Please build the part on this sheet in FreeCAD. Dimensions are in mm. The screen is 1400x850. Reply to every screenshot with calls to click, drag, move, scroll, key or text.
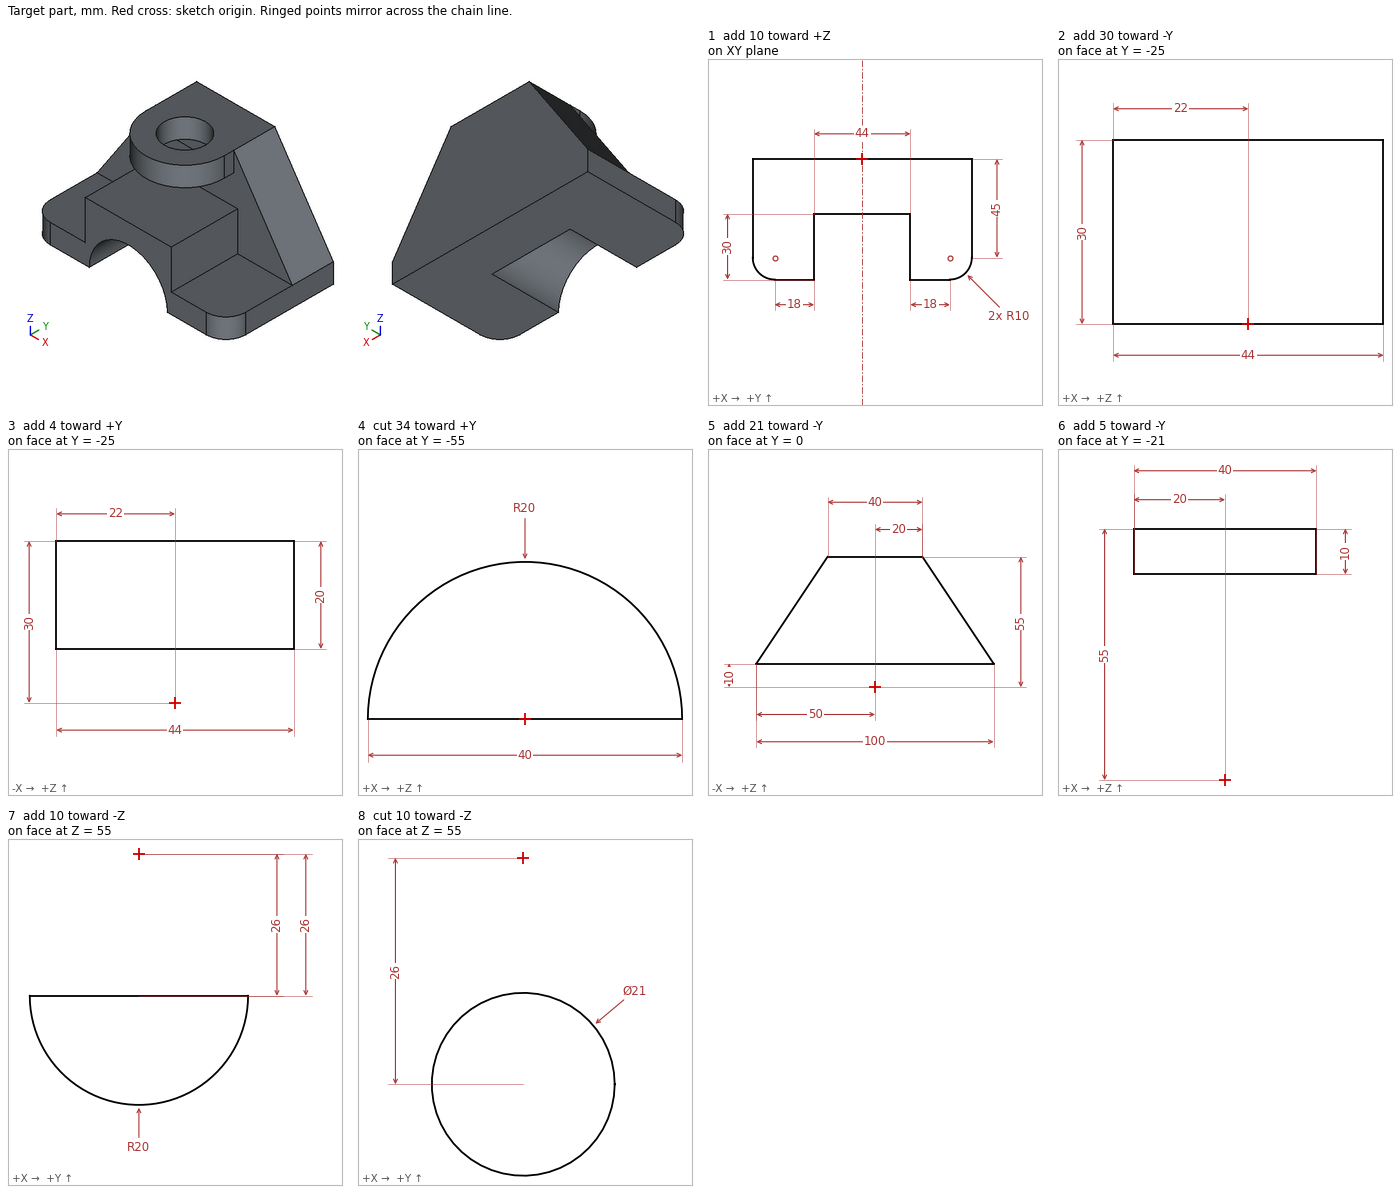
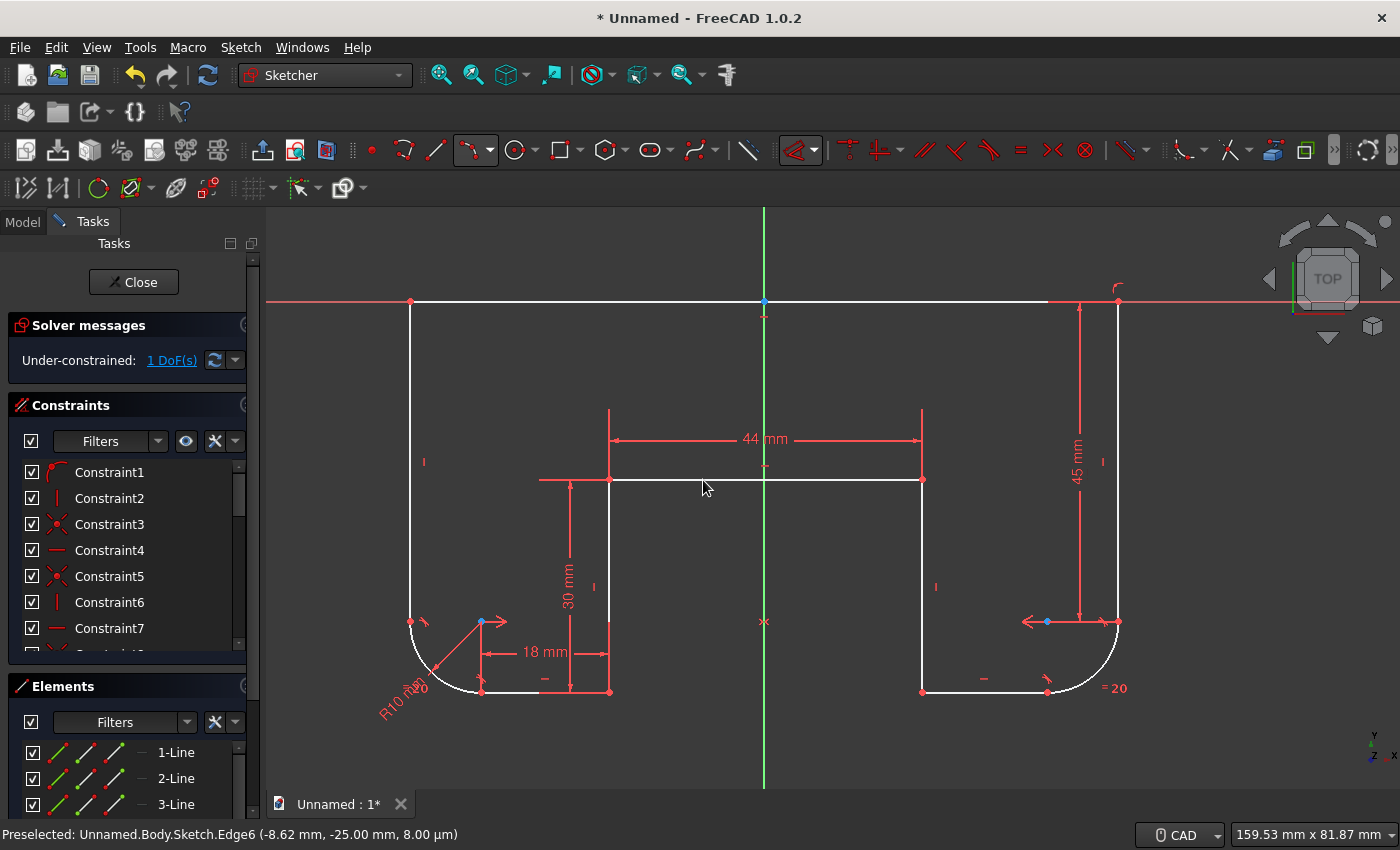
click(960, 693)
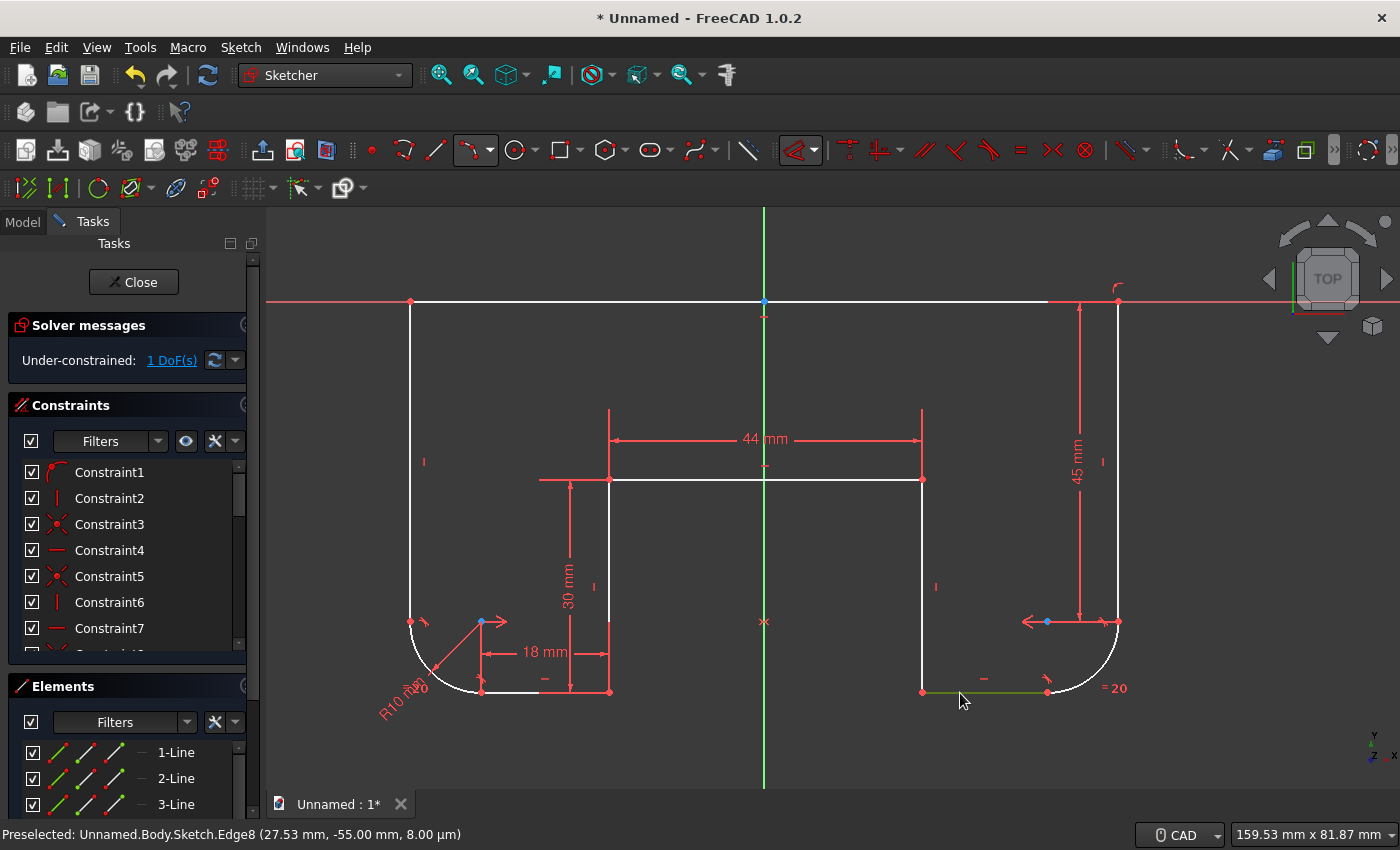
key(l)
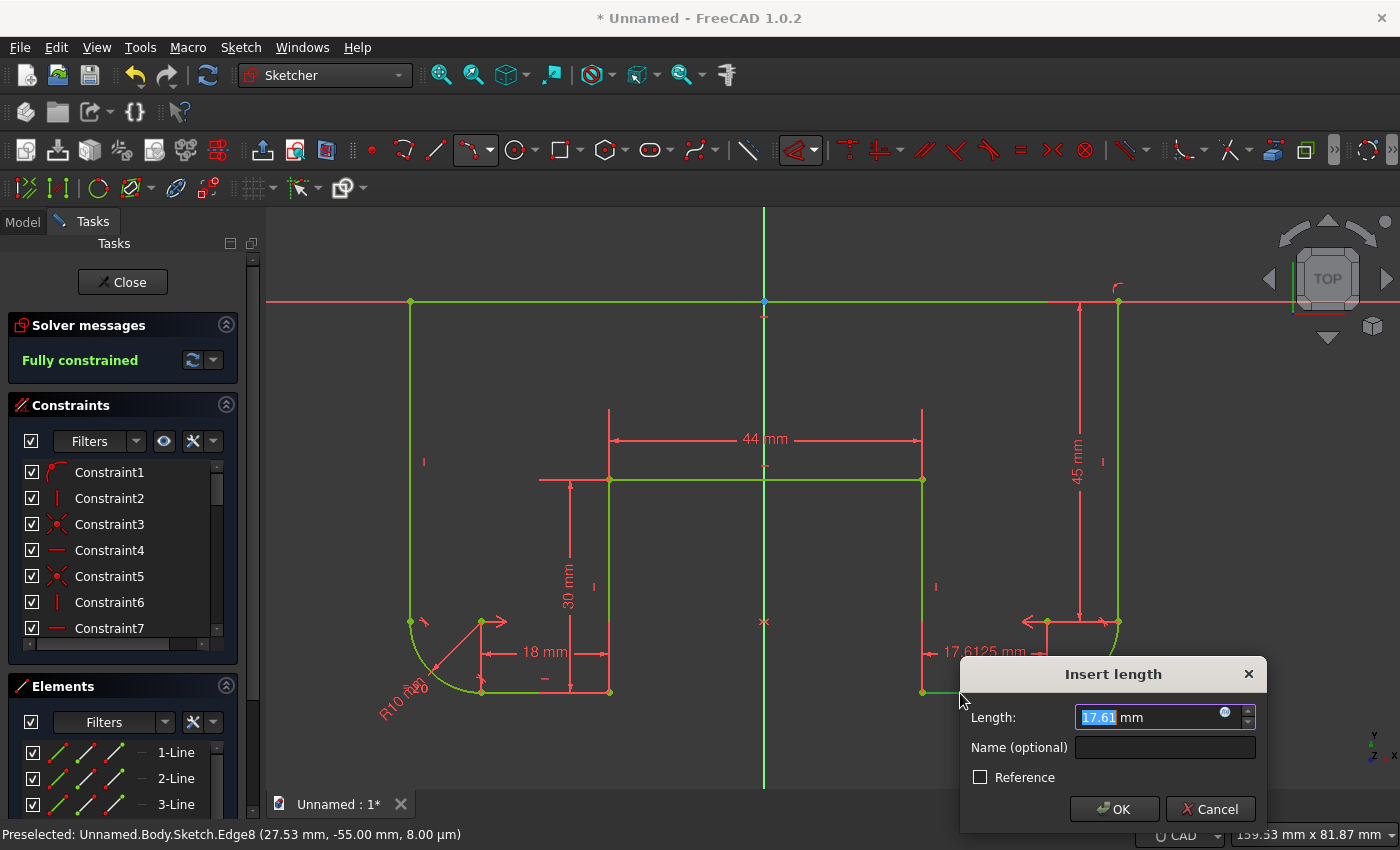
text(18)
key(Return)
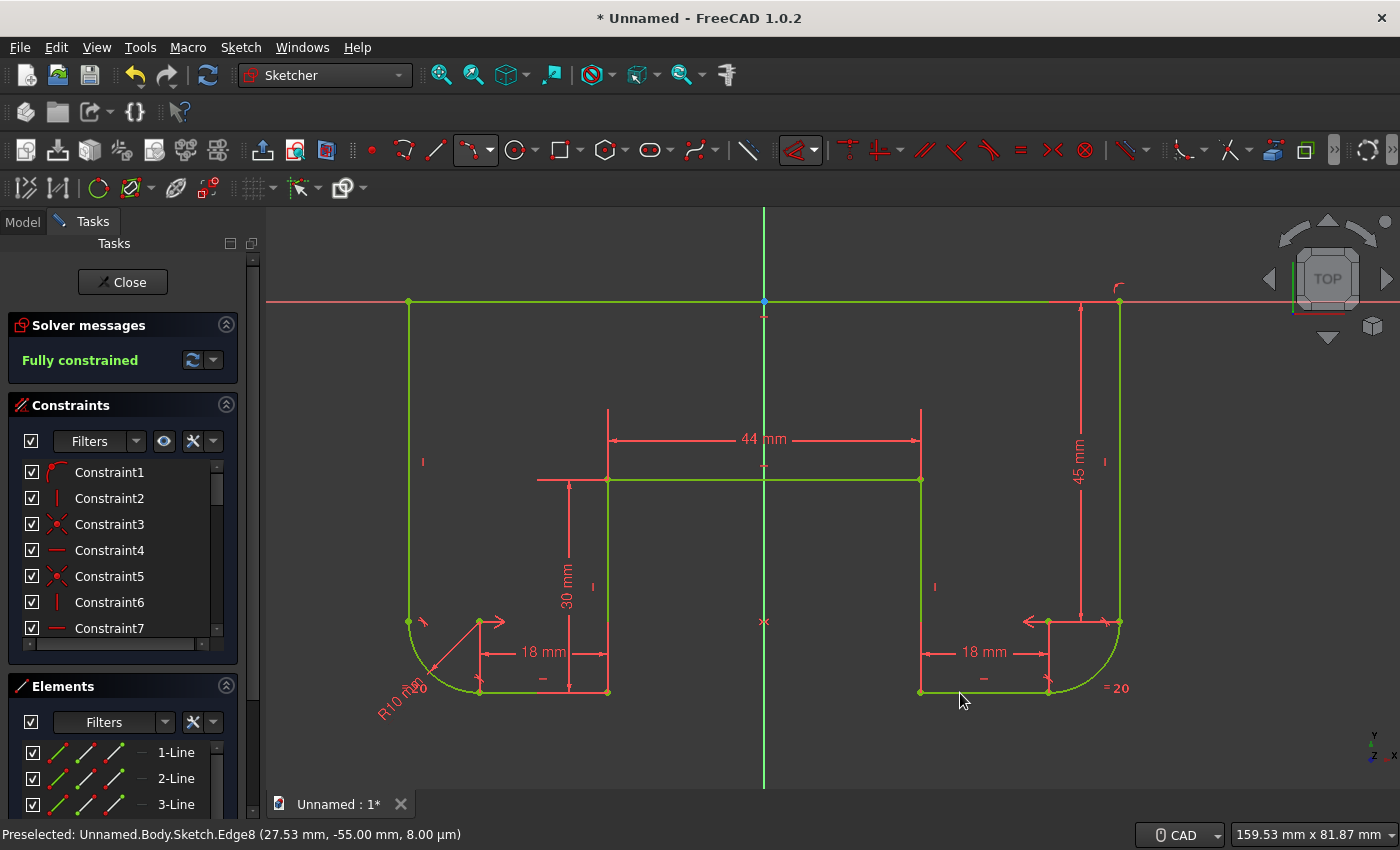
click(123, 282)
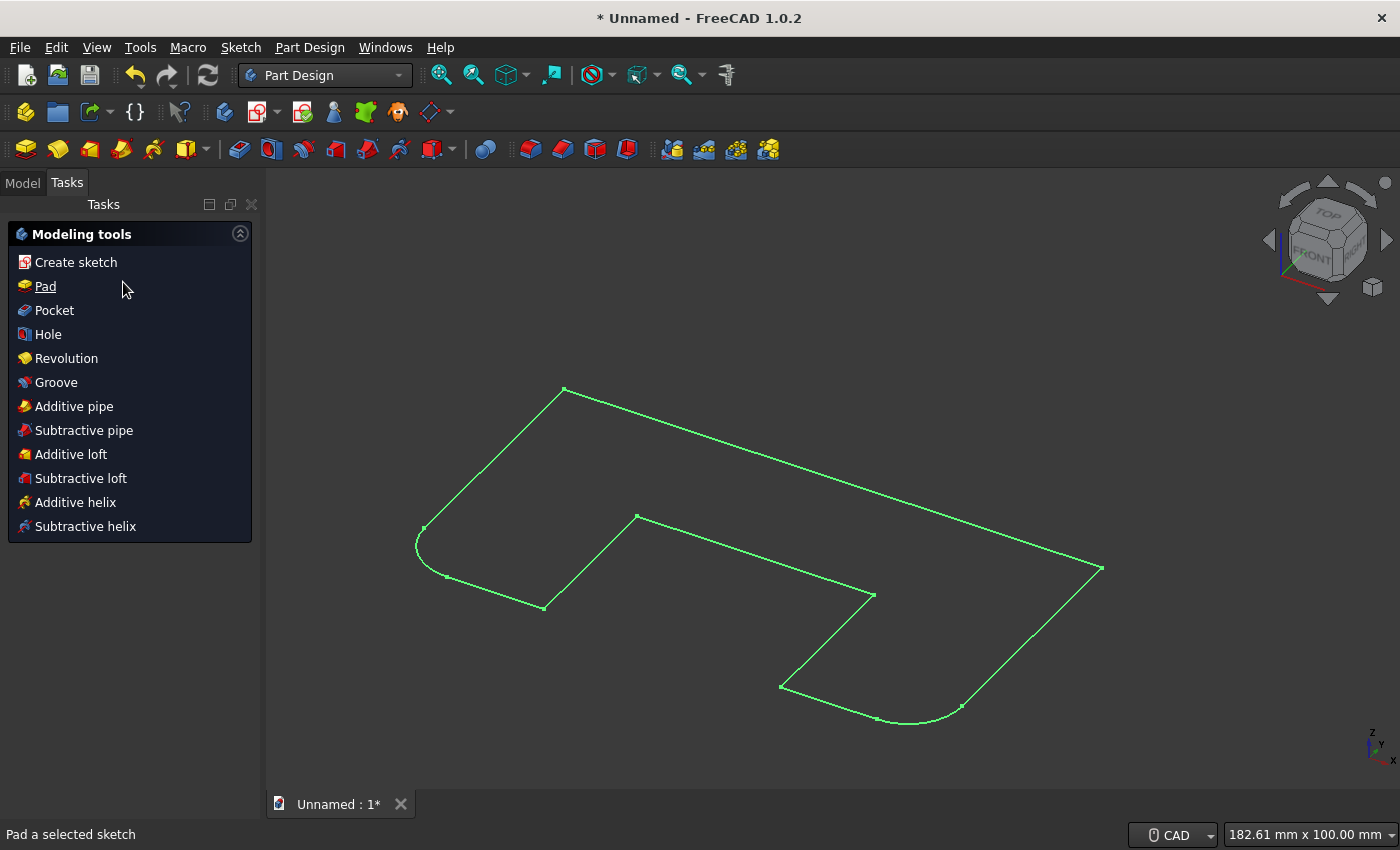
click(26, 150)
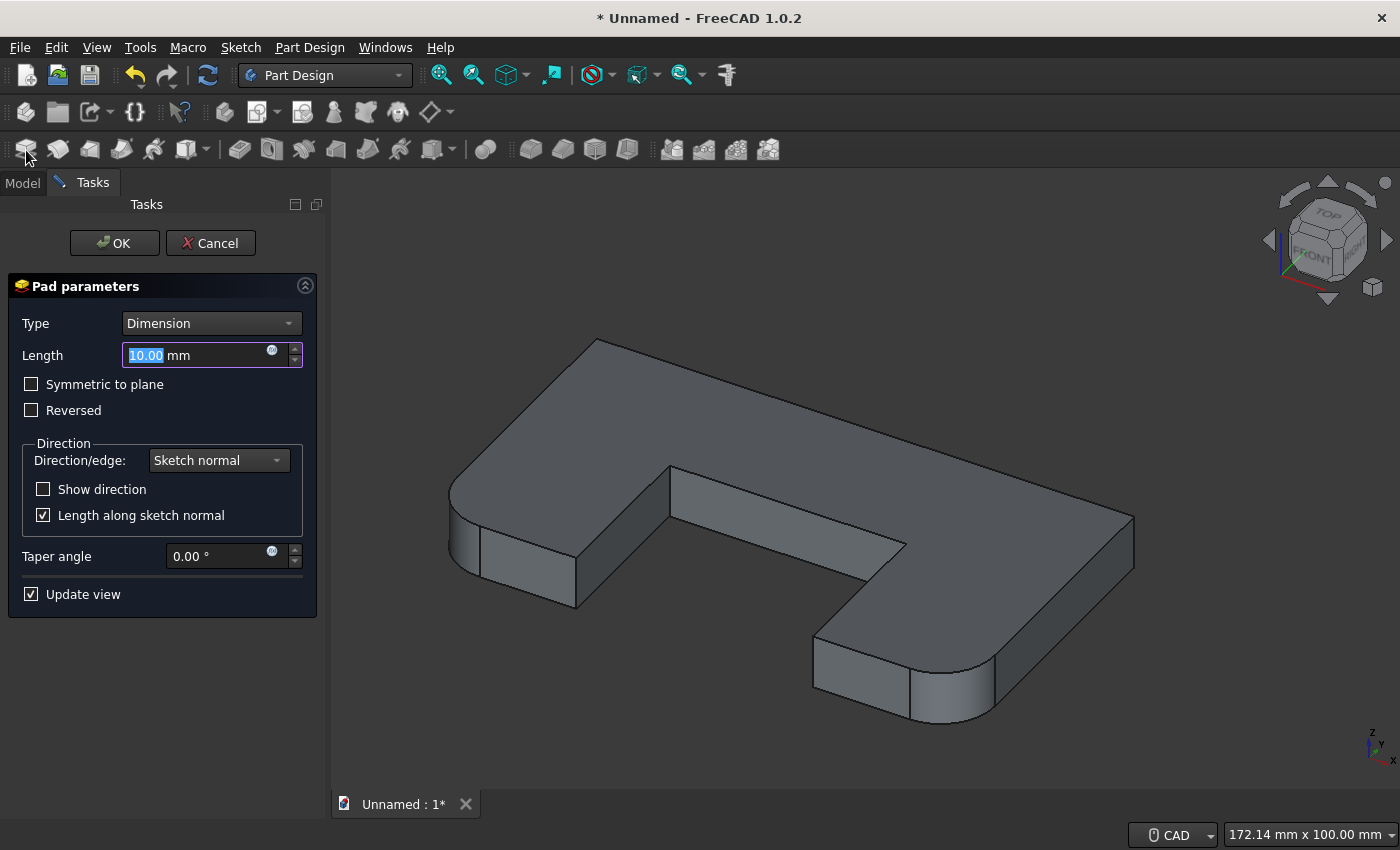
text(10)
key(Tab)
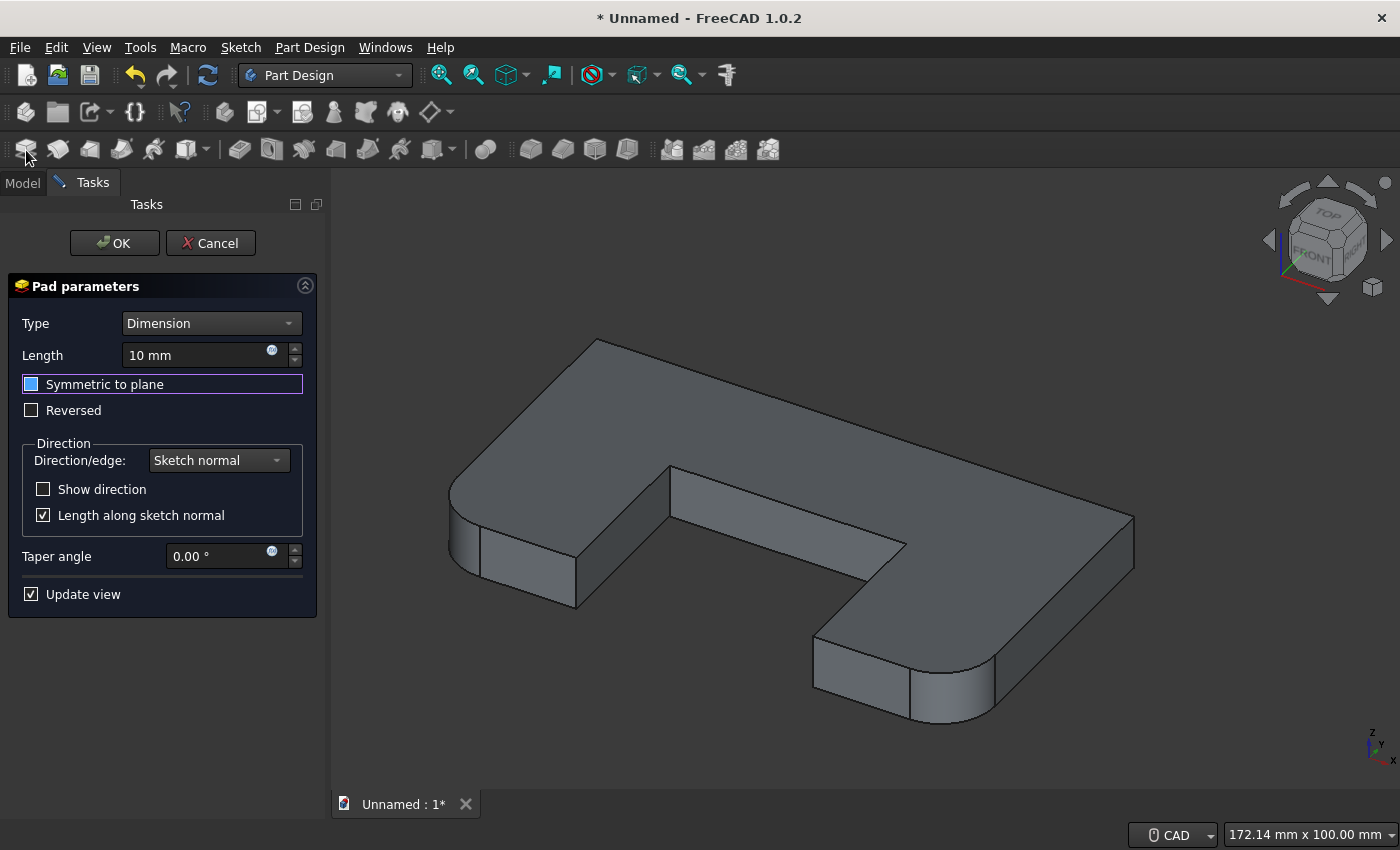
click(115, 243)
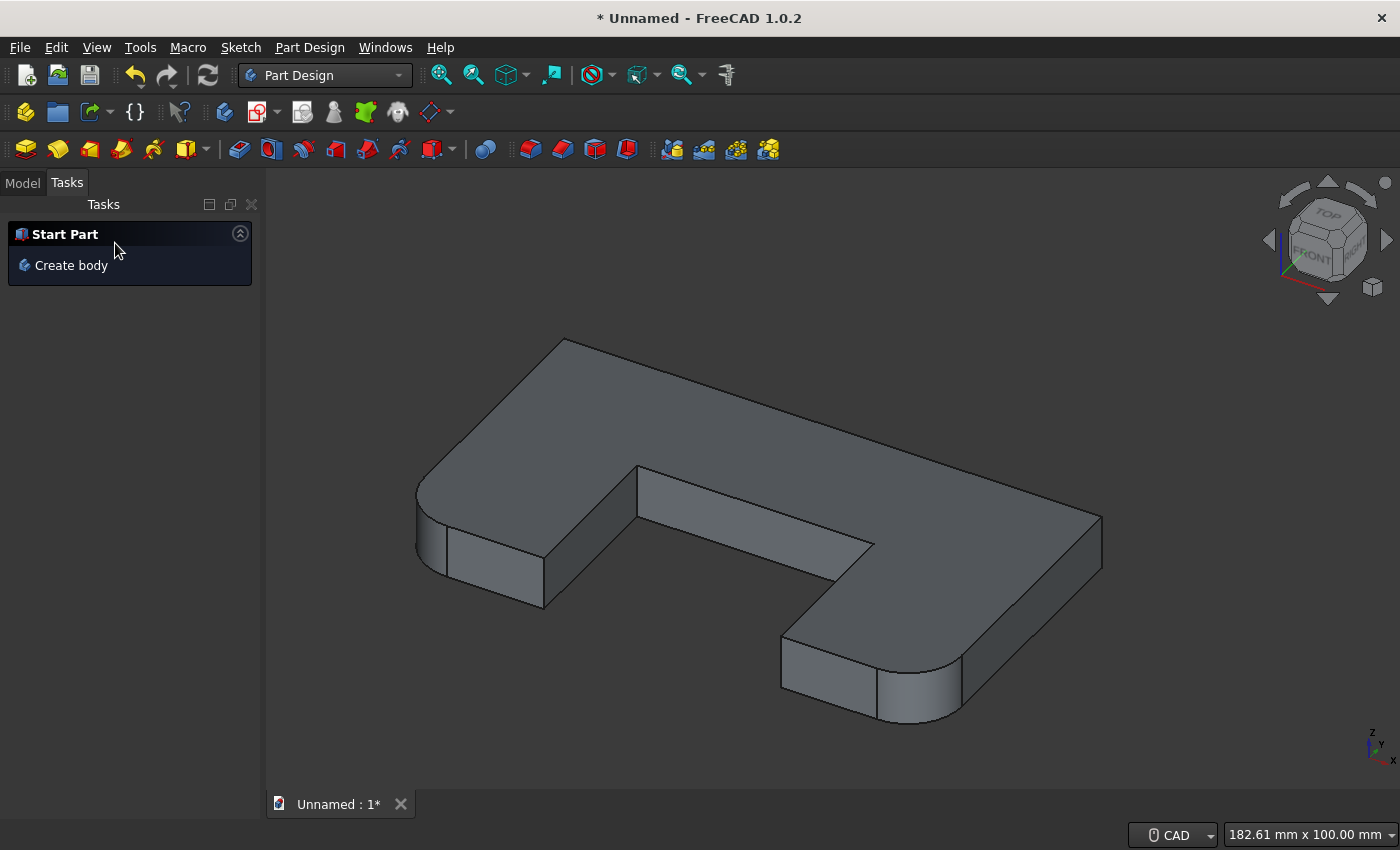
click(823, 552)